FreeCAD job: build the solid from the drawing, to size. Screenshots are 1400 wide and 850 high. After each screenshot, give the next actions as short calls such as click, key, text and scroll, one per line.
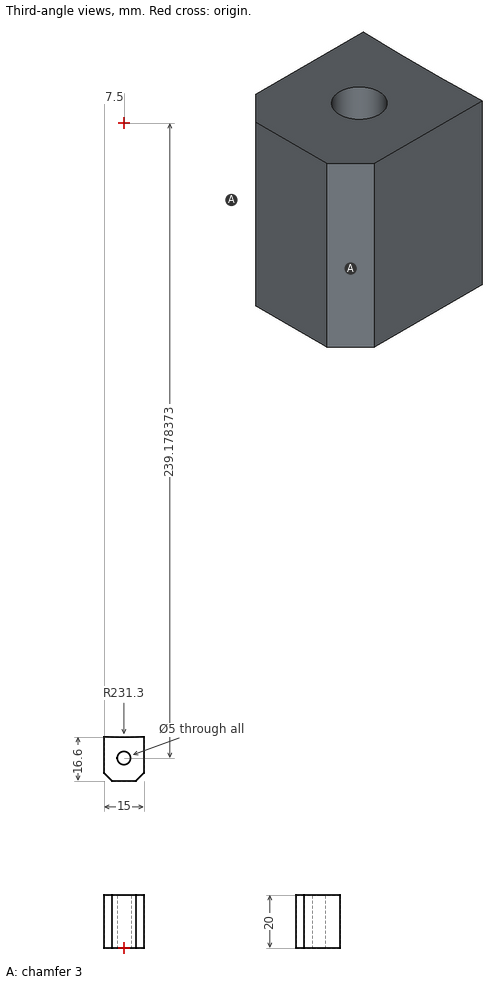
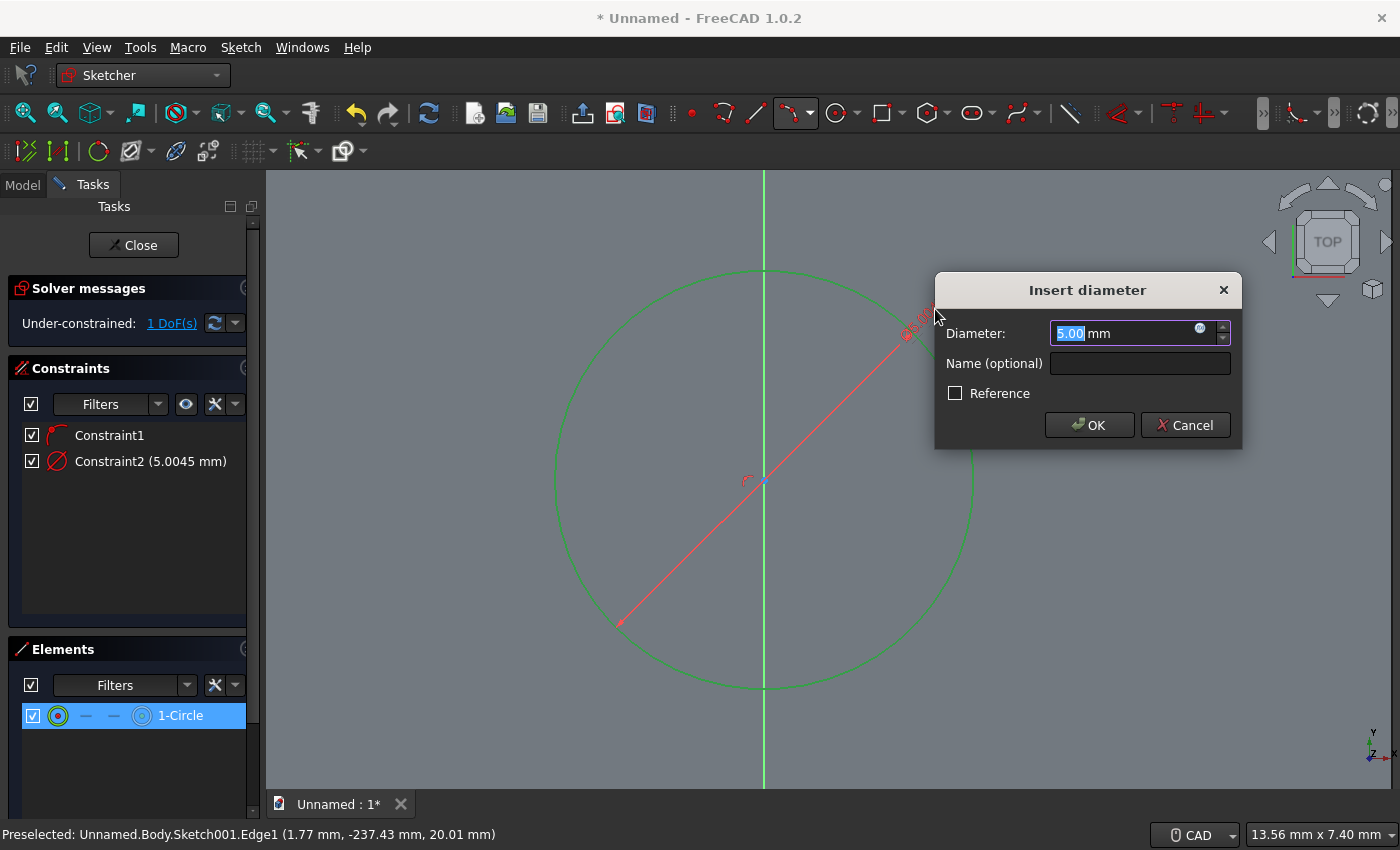
text(5)
key(Return)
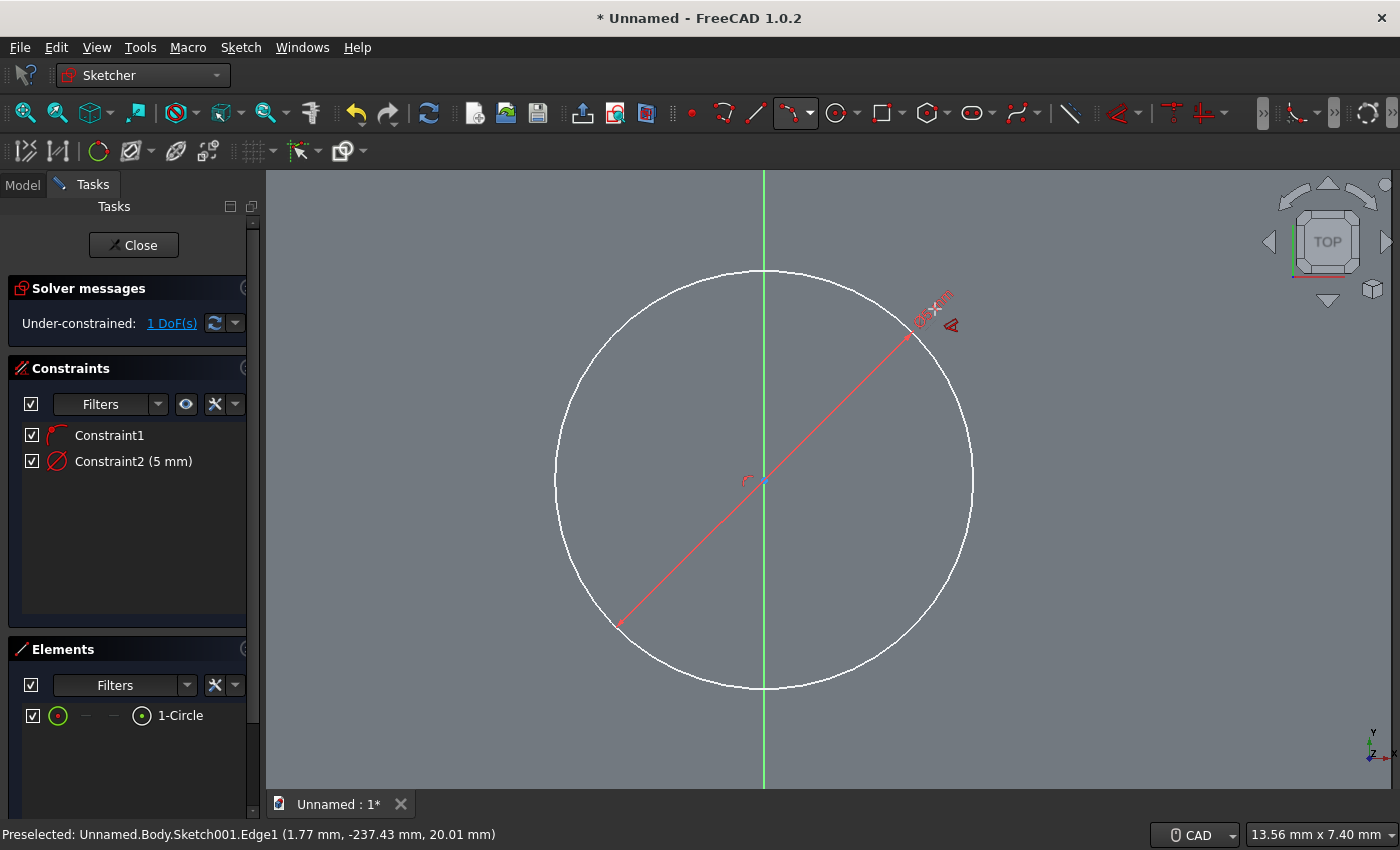
click(764, 480)
click(798, 339)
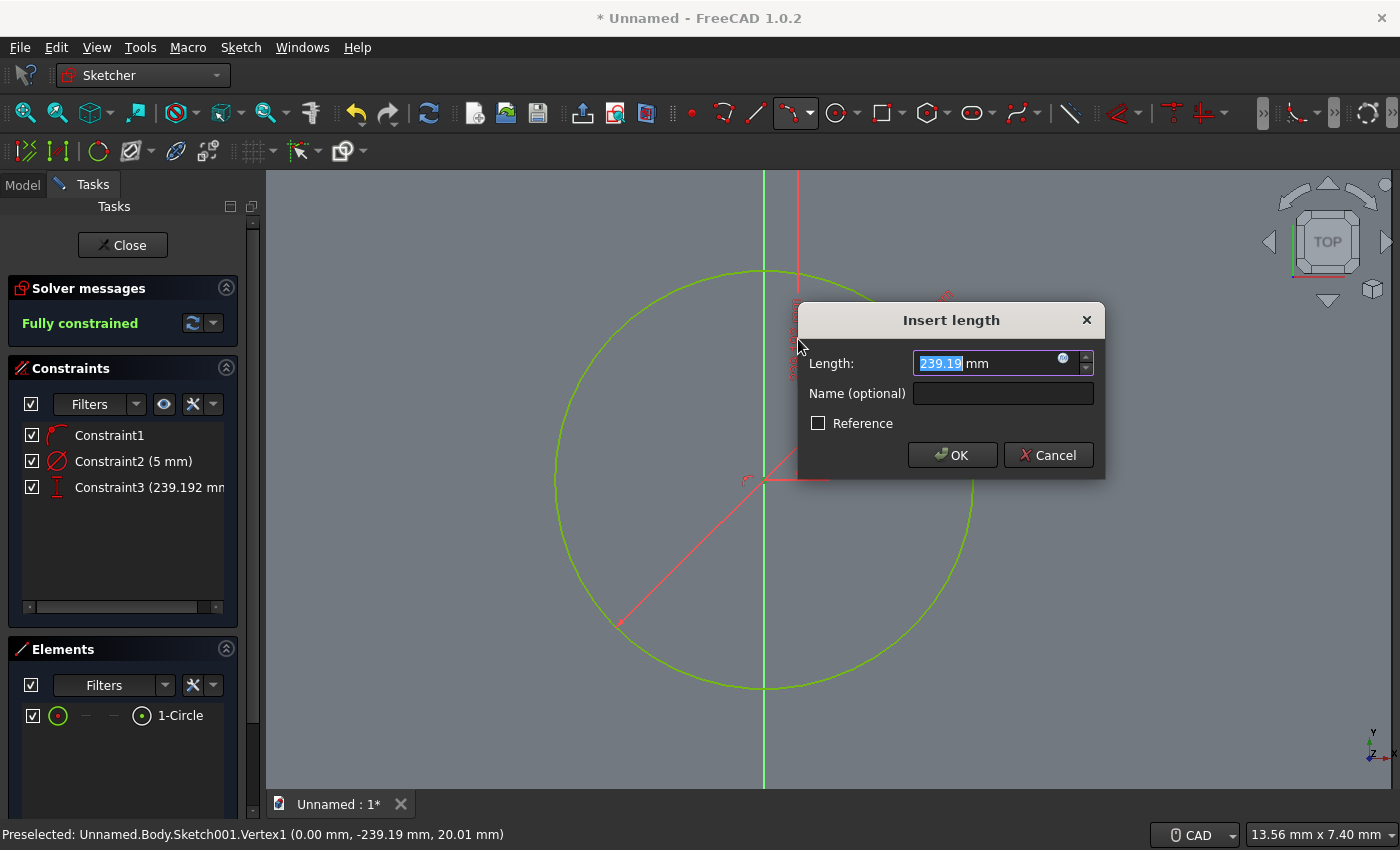
text(239.178373)
key(Return)
key(Escape)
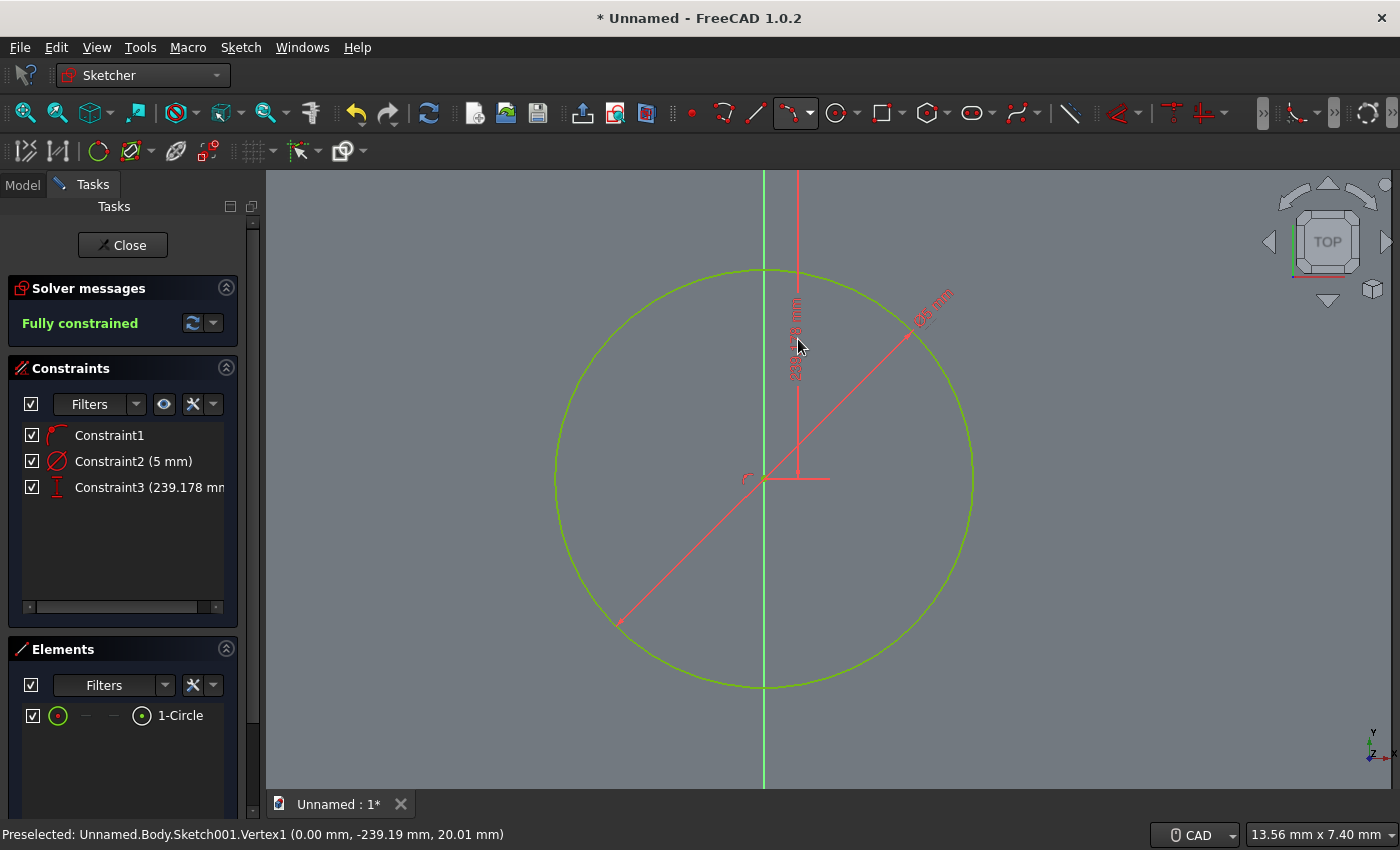
click(123, 245)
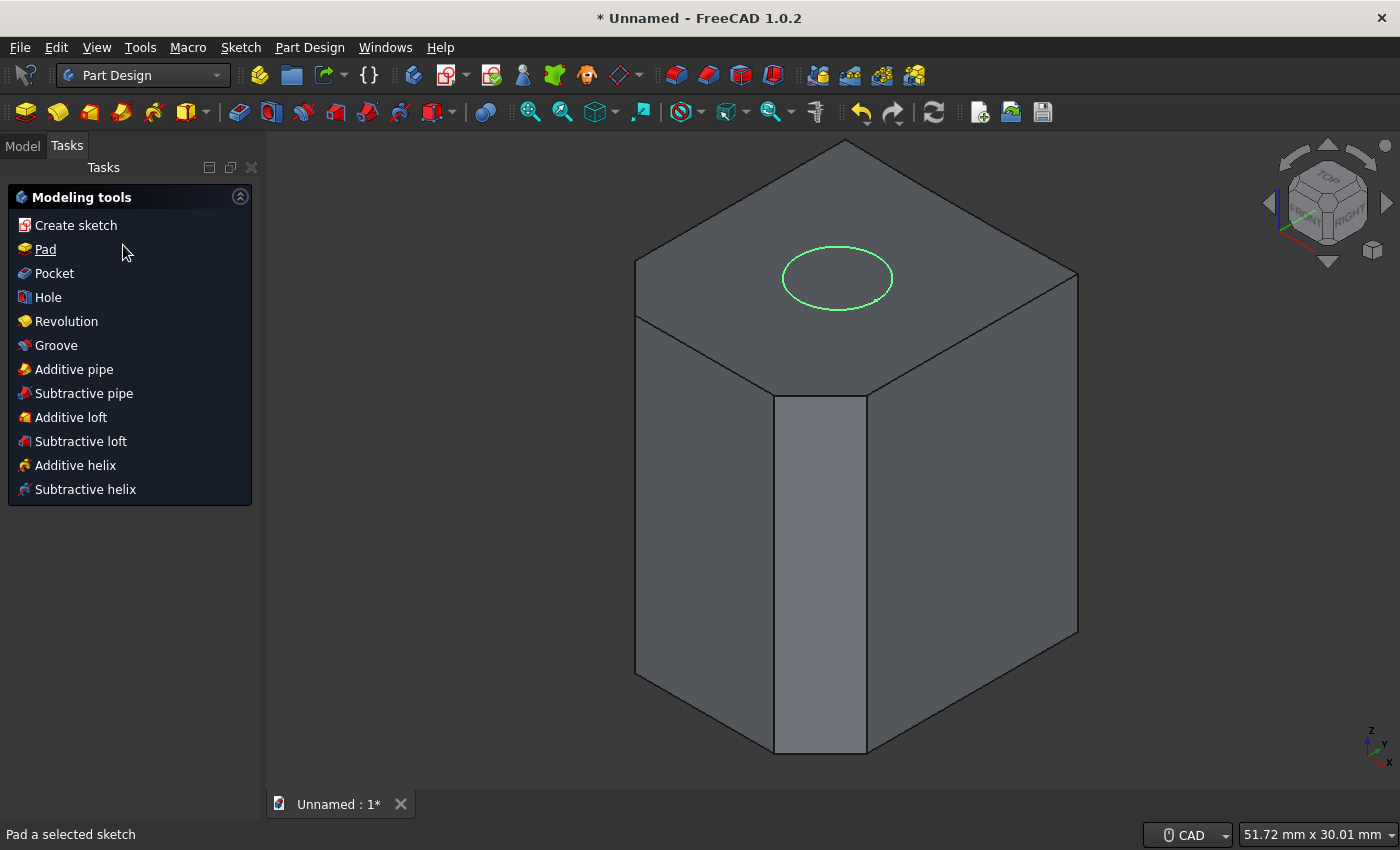
click(272, 112)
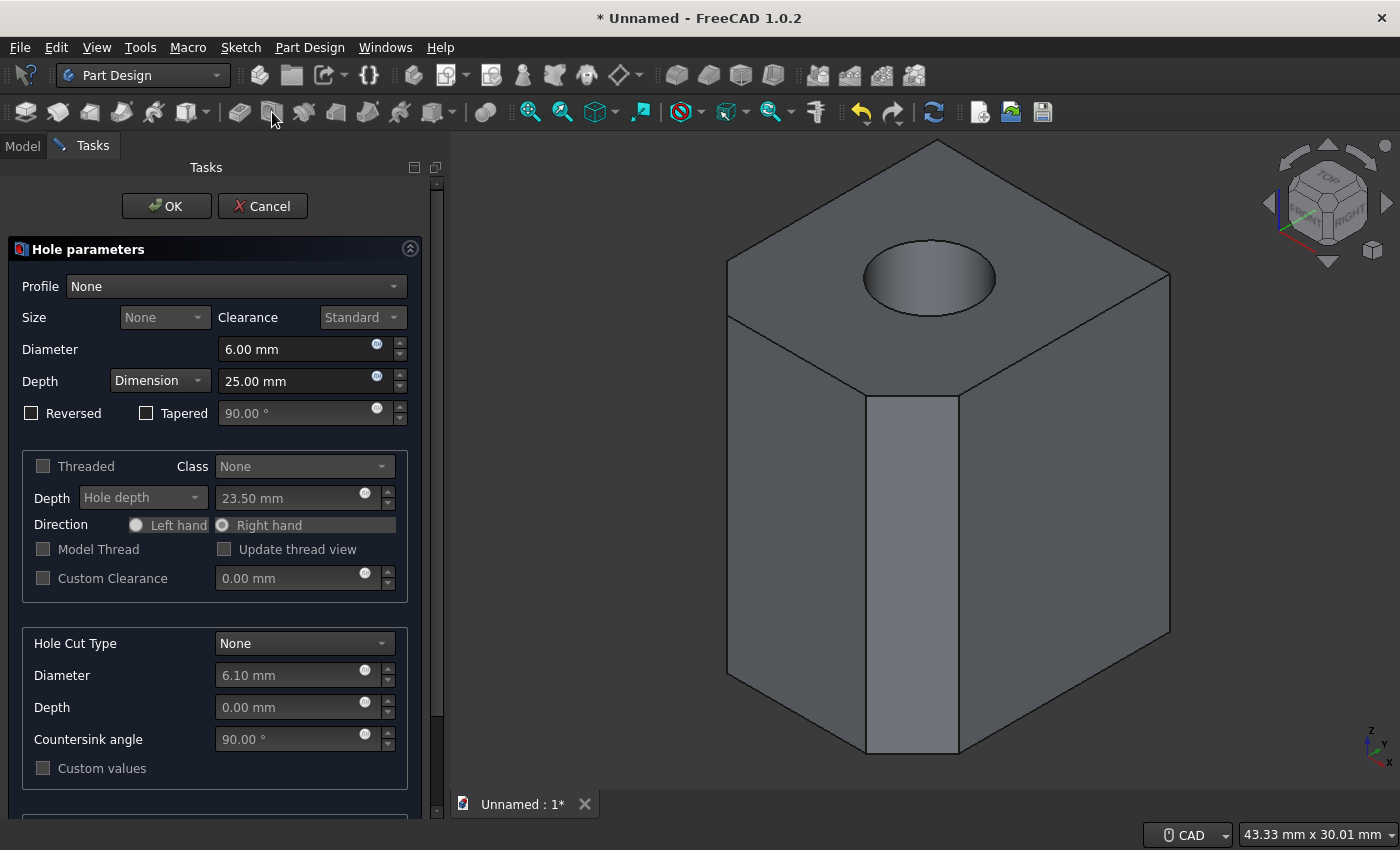
triple_click(305, 349)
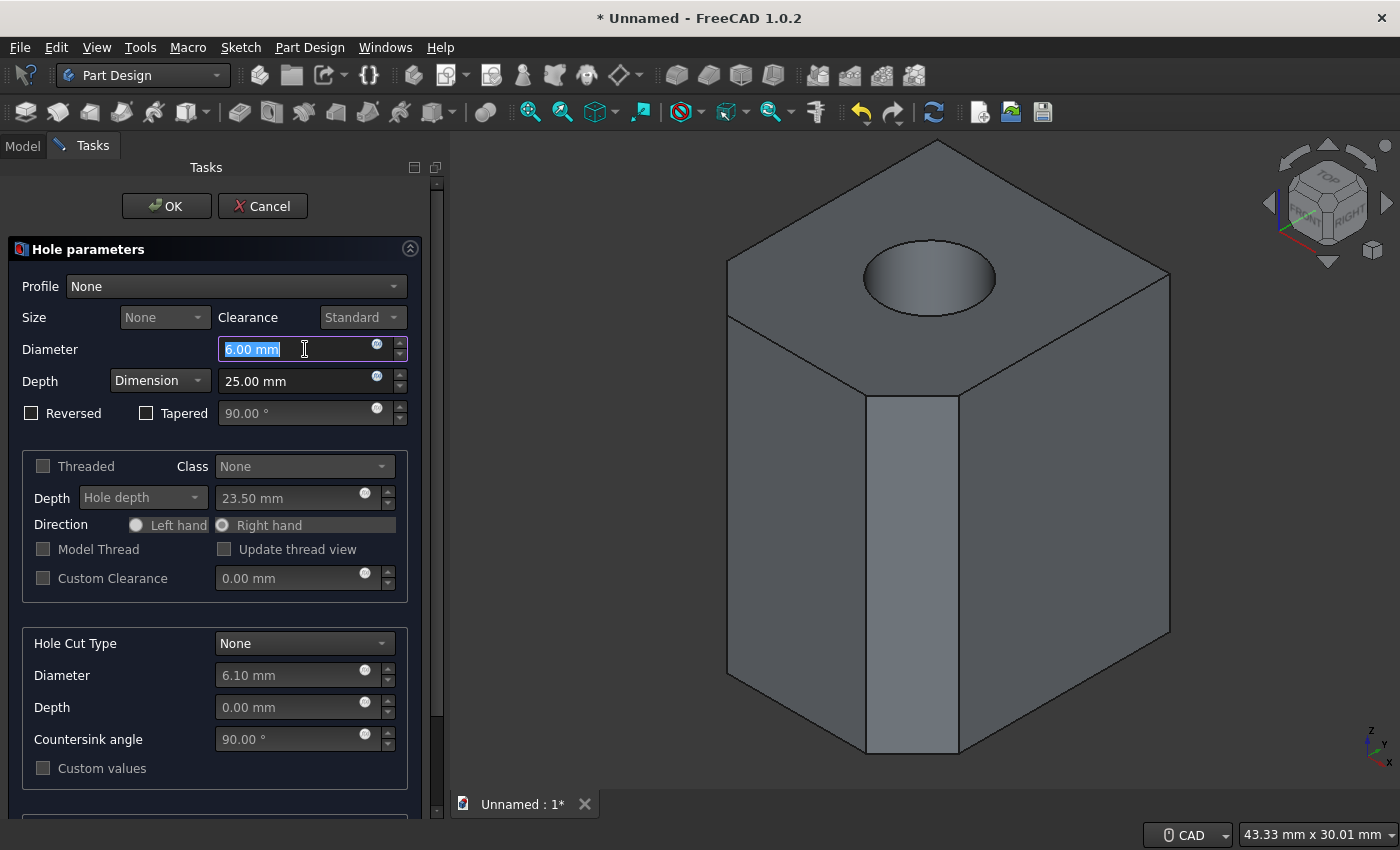
text(5)
key(Tab)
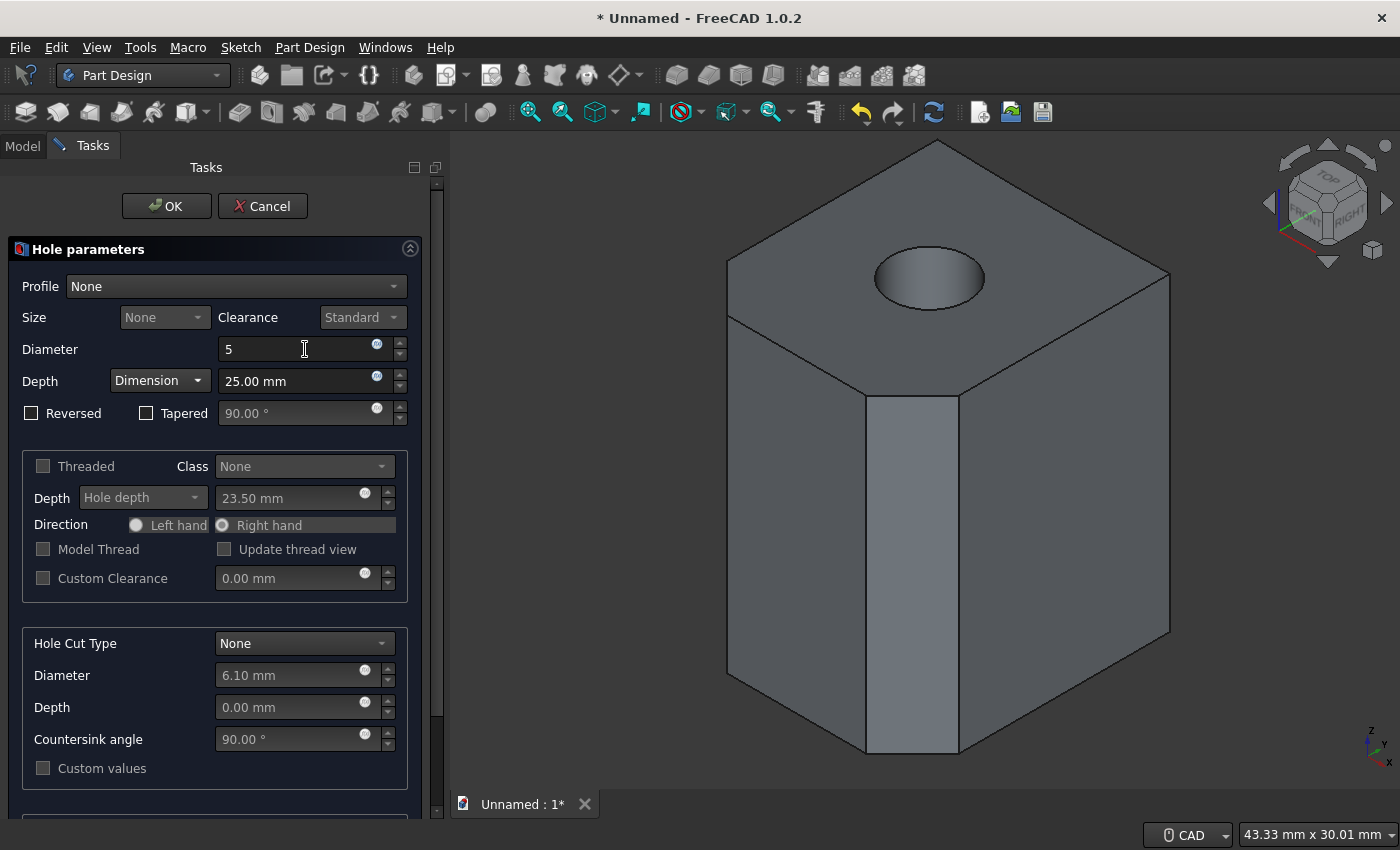
click(161, 380)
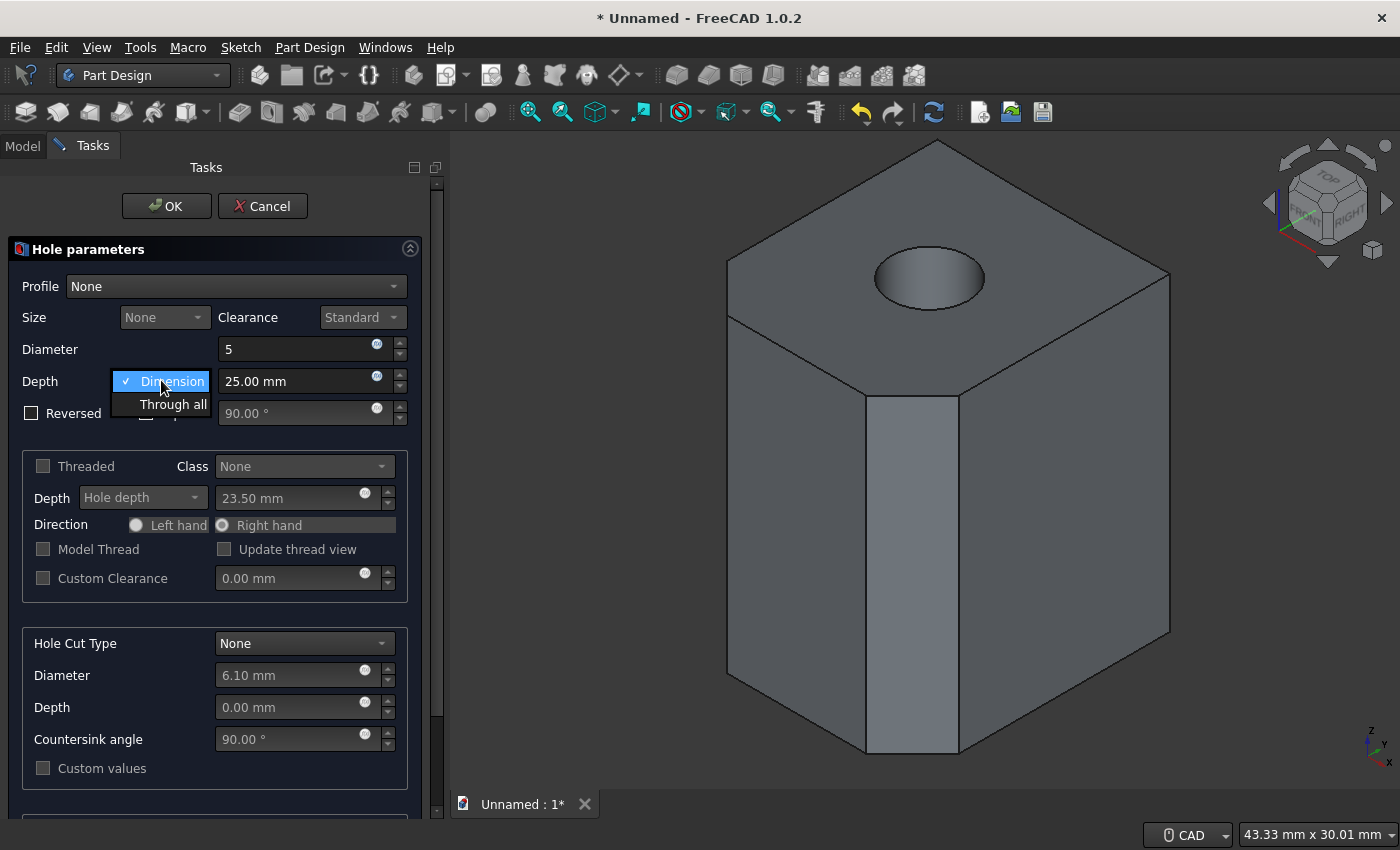
click(160, 404)